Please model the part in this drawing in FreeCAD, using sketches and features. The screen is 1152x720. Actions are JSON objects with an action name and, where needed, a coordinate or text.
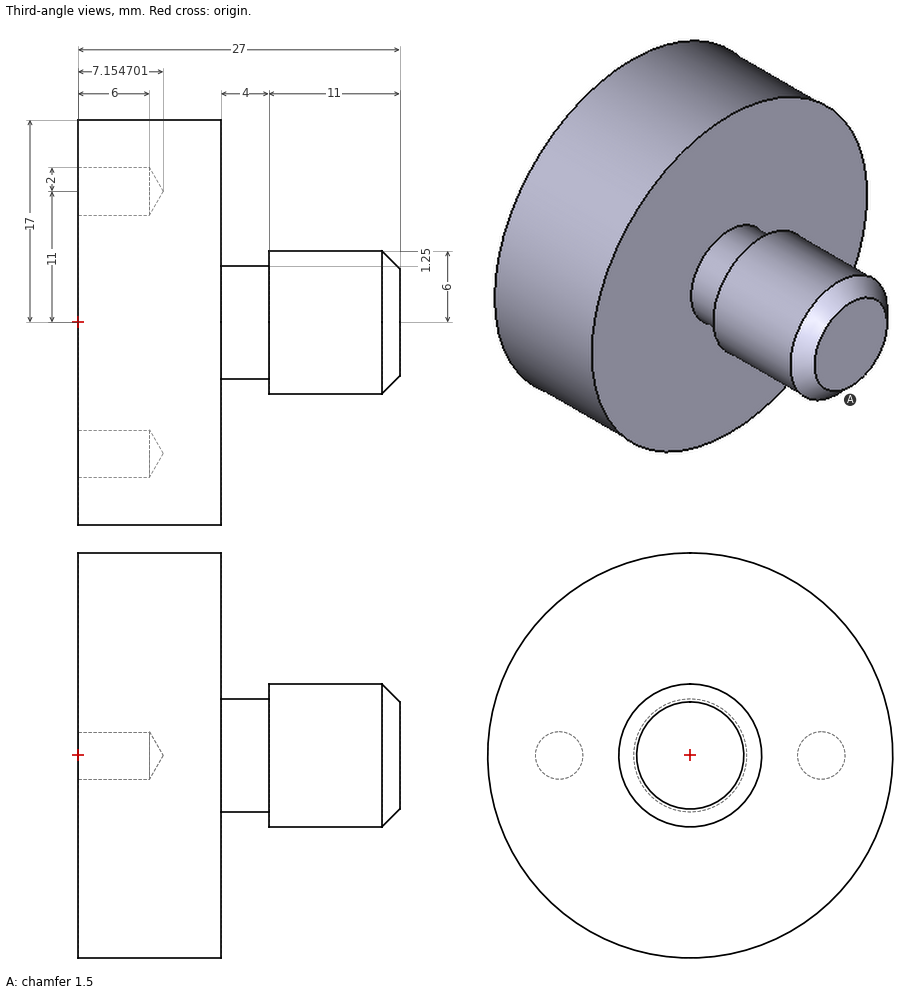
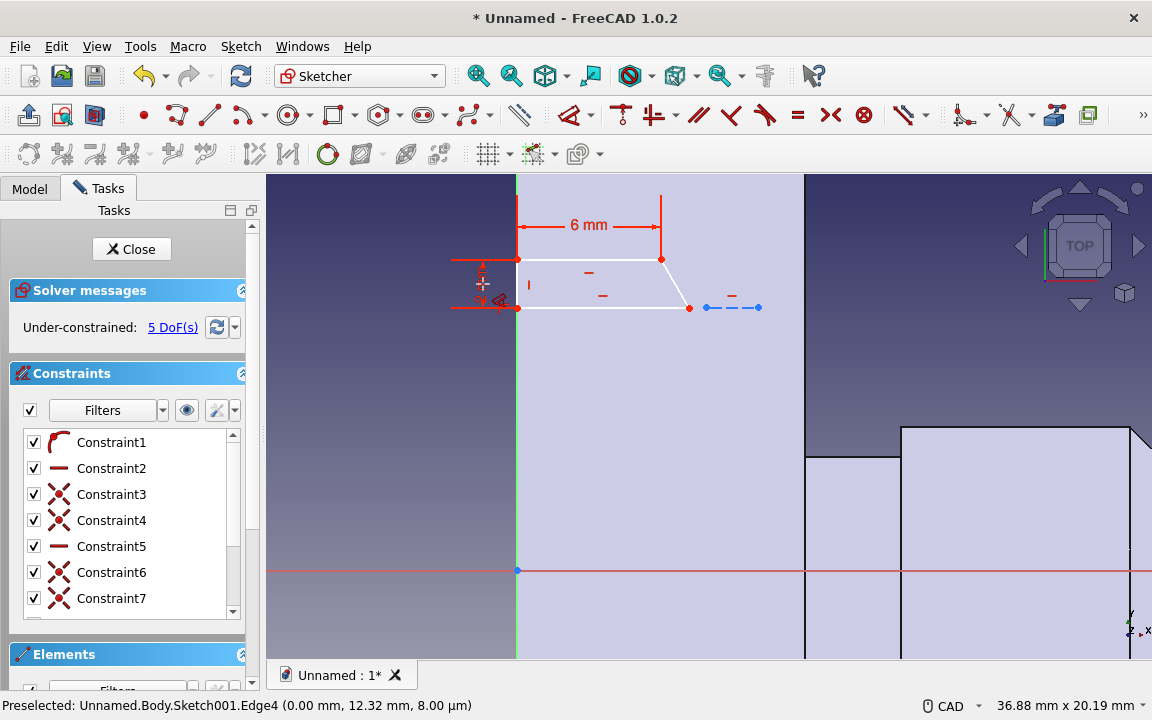
{"action": "left_click", "coordinate": [517, 308]}
{"action": "left_click", "coordinate": [483, 440]}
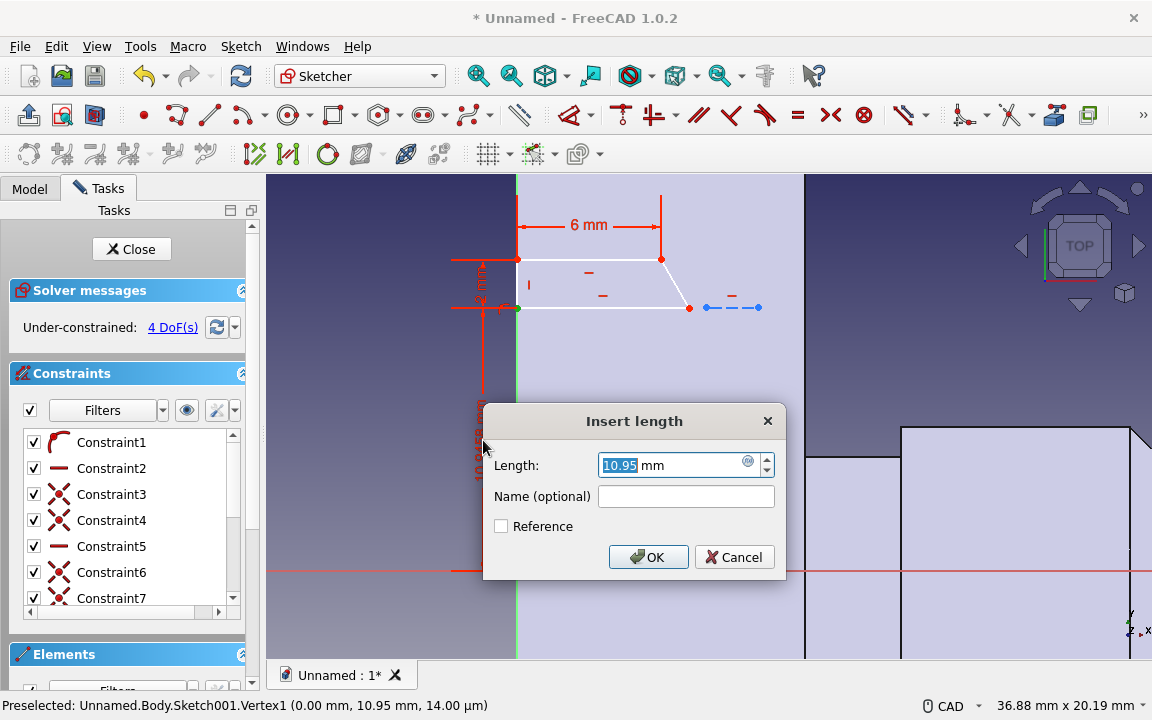
{"action": "type", "text": "11"}
{"action": "key", "text": "Return"}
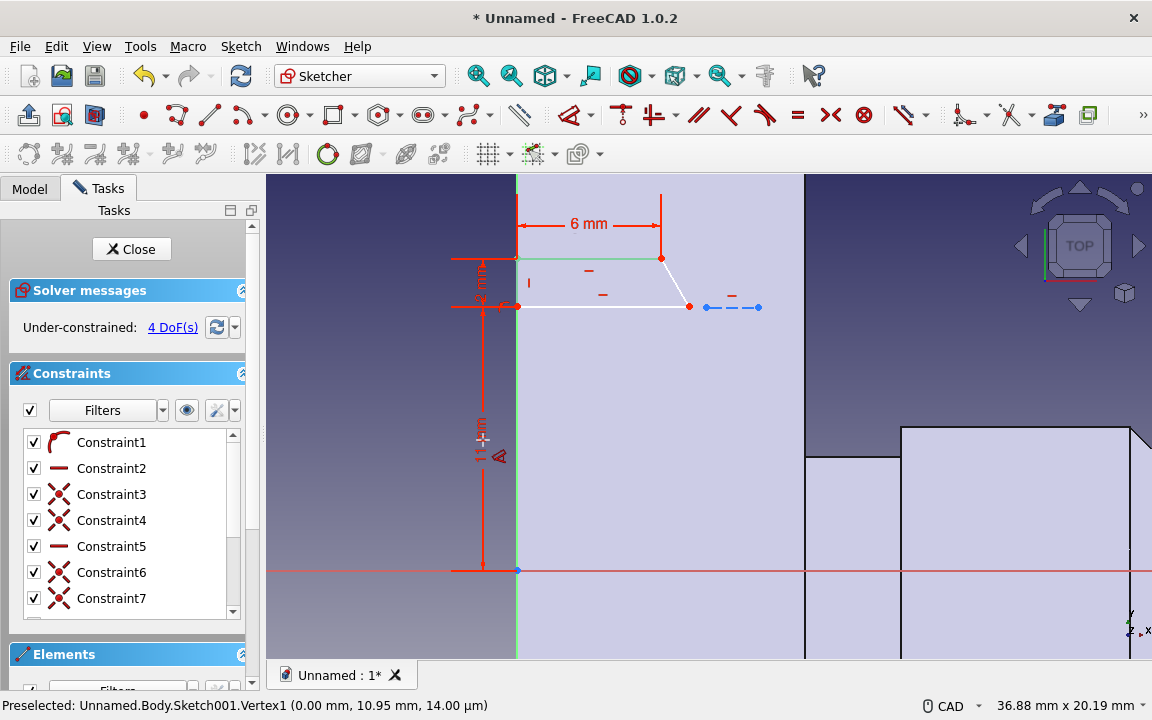
{"action": "left_click", "coordinate": [706, 308]}
{"action": "left_click", "coordinate": [483, 379]}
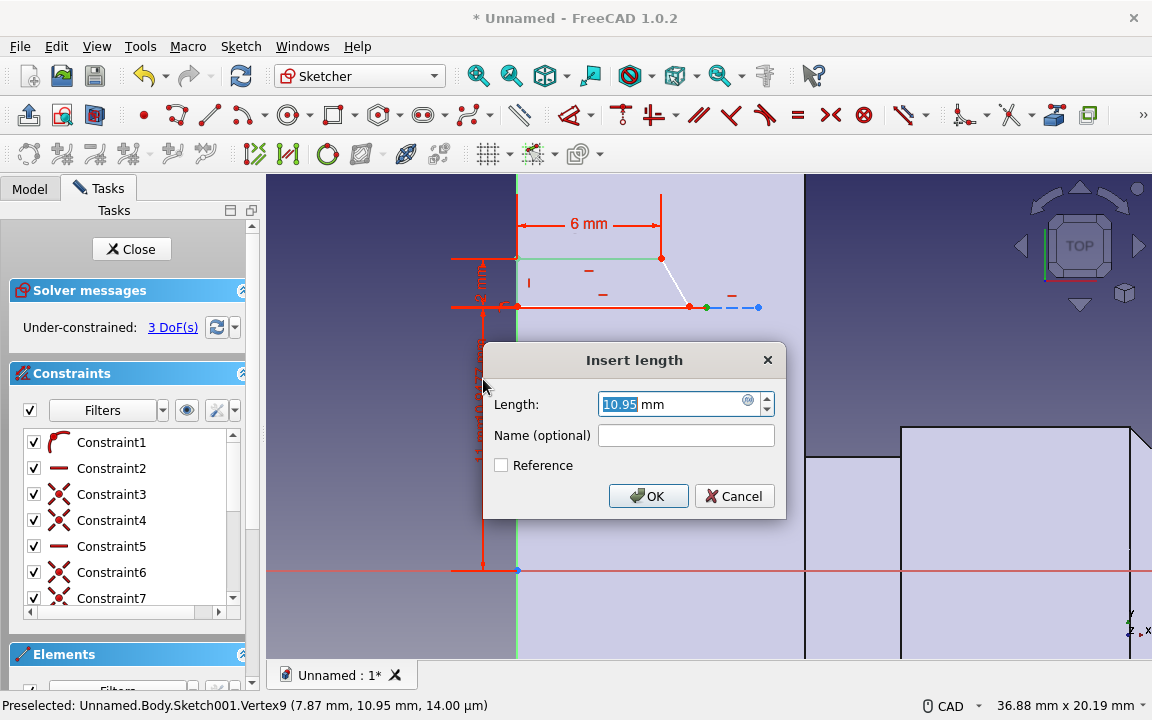
{"action": "type", "text": "11"}
{"action": "key", "text": "Return"}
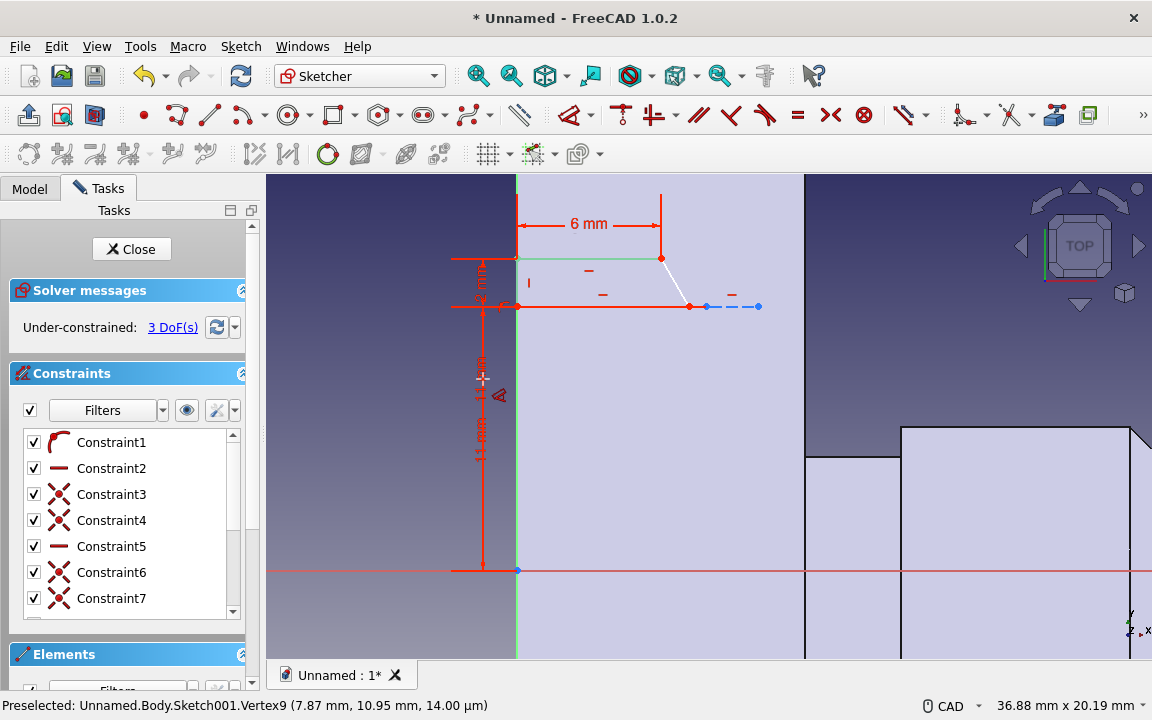
{"action": "left_click", "coordinate": [569, 307]}
{"action": "left_click", "coordinate": [603, 273]}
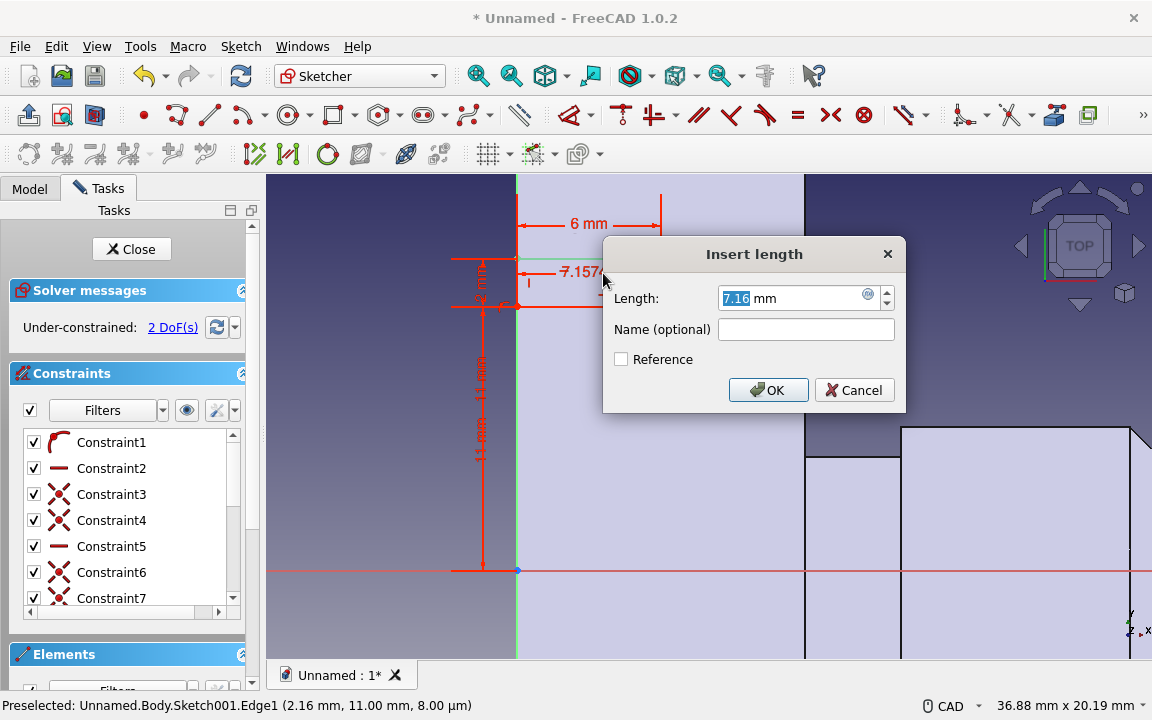
{"action": "type", "text": "7.154701"}
{"action": "key", "text": "Return"}
{"action": "key", "text": "Escape"}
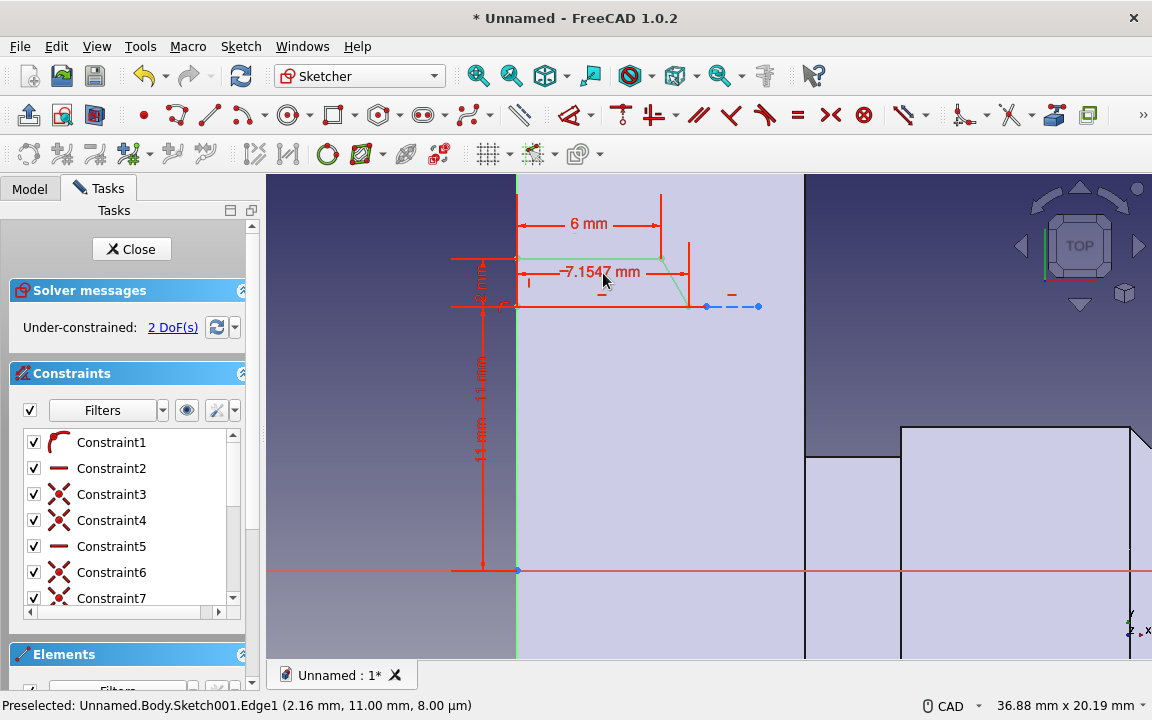
{"action": "left_click", "coordinate": [132, 249]}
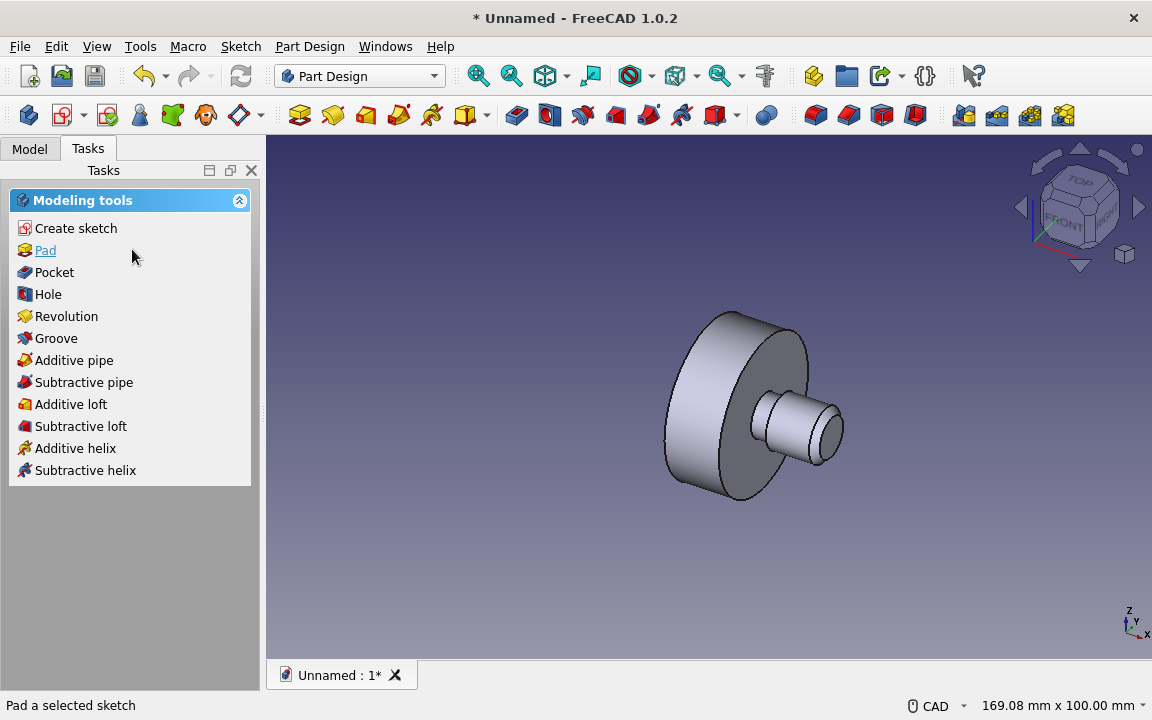
{"action": "left_click", "coordinate": [583, 116]}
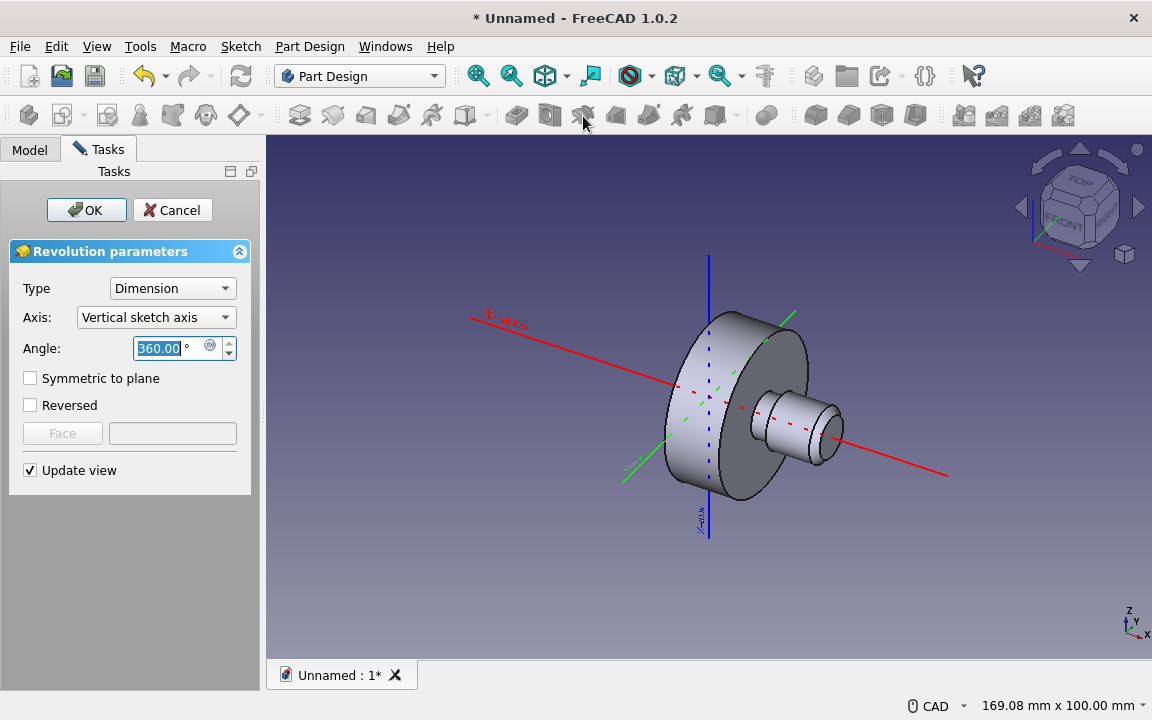
{"action": "left_click", "coordinate": [157, 318]}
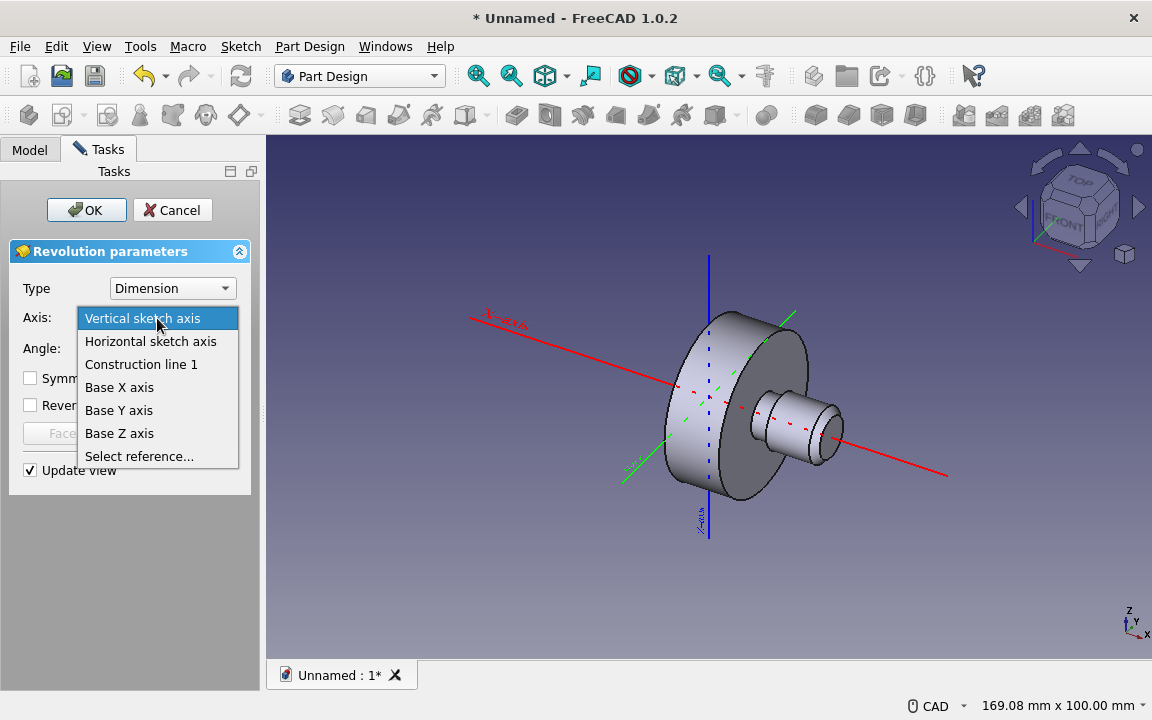
{"action": "left_click", "coordinate": [156, 364]}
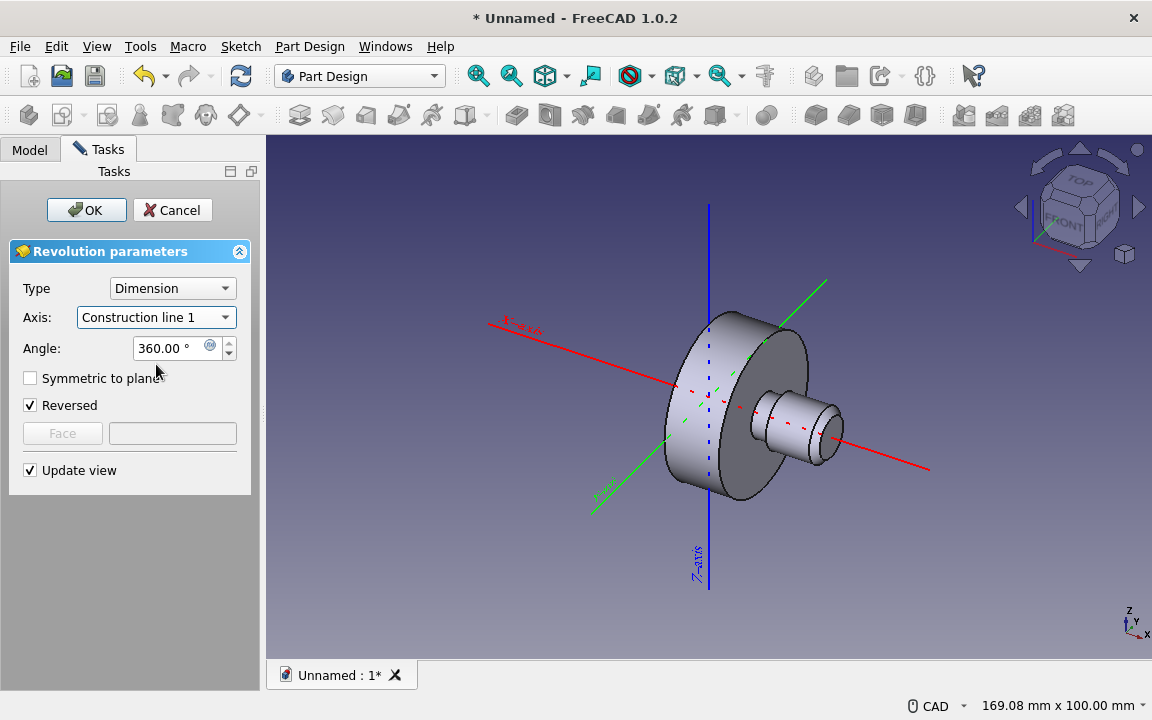
{"action": "left_click", "coordinate": [87, 210]}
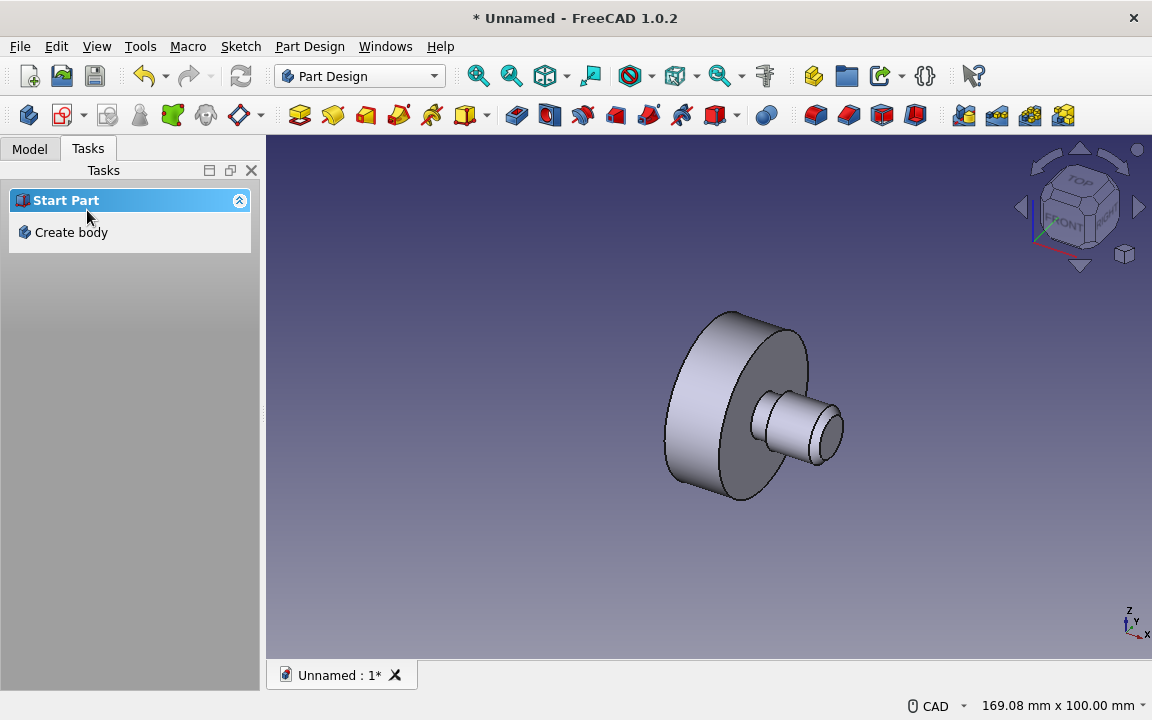
{"action": "left_click", "coordinate": [30, 148]}